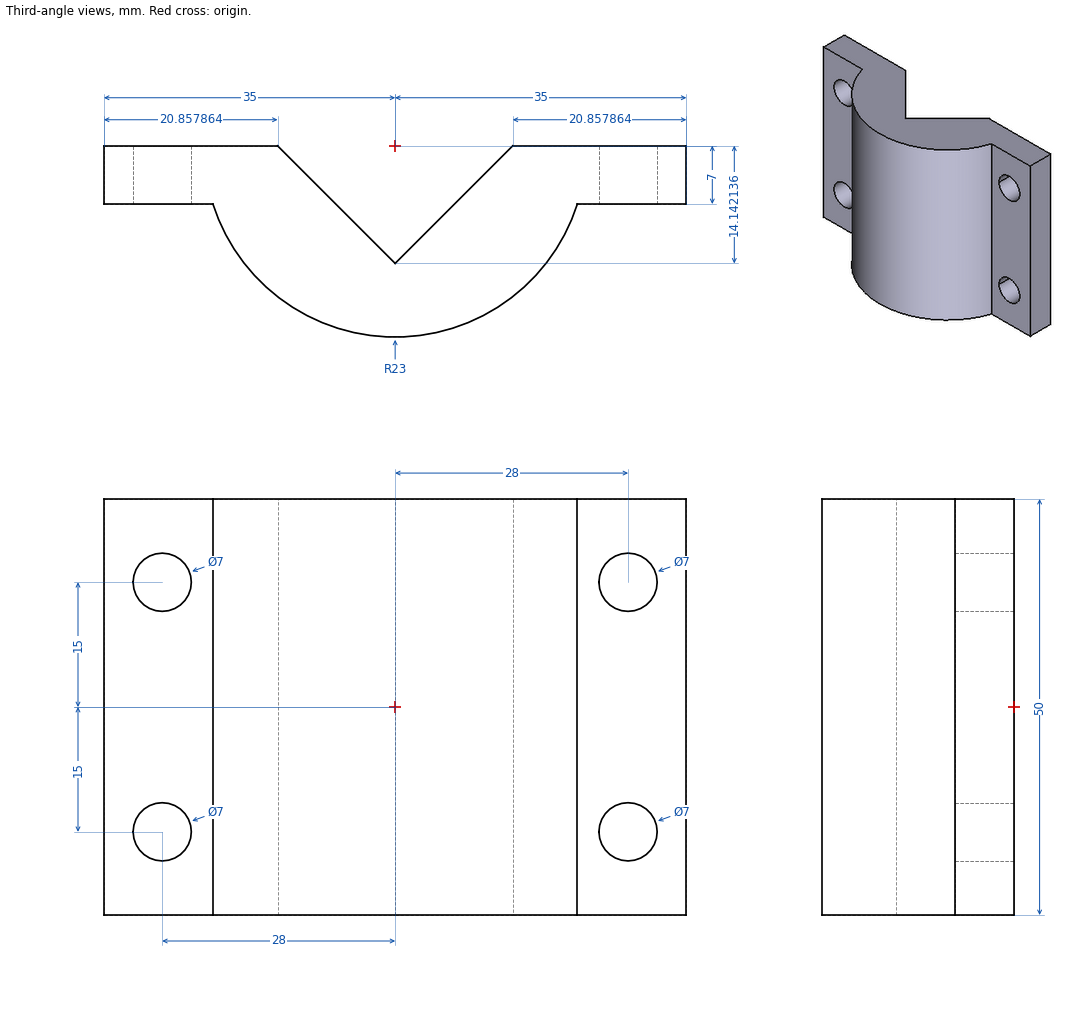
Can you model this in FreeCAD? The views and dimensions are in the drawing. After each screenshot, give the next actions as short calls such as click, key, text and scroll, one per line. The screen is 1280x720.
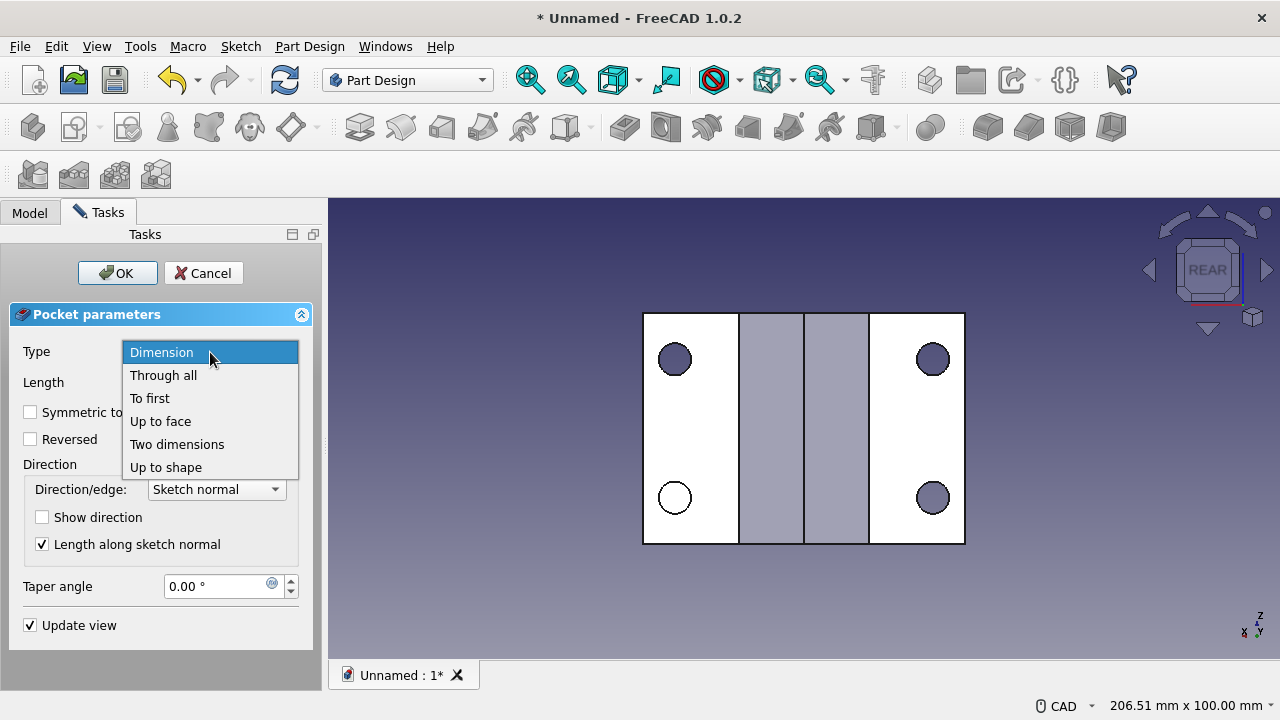
click(208, 398)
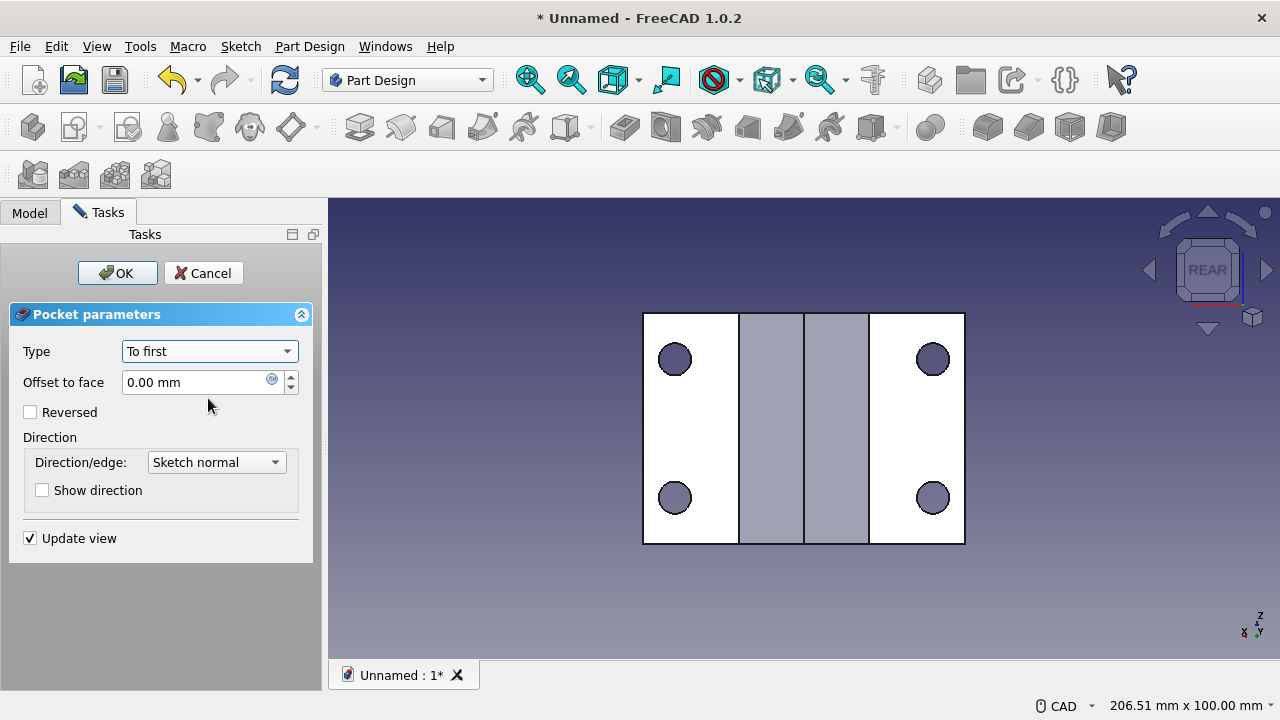
click(118, 273)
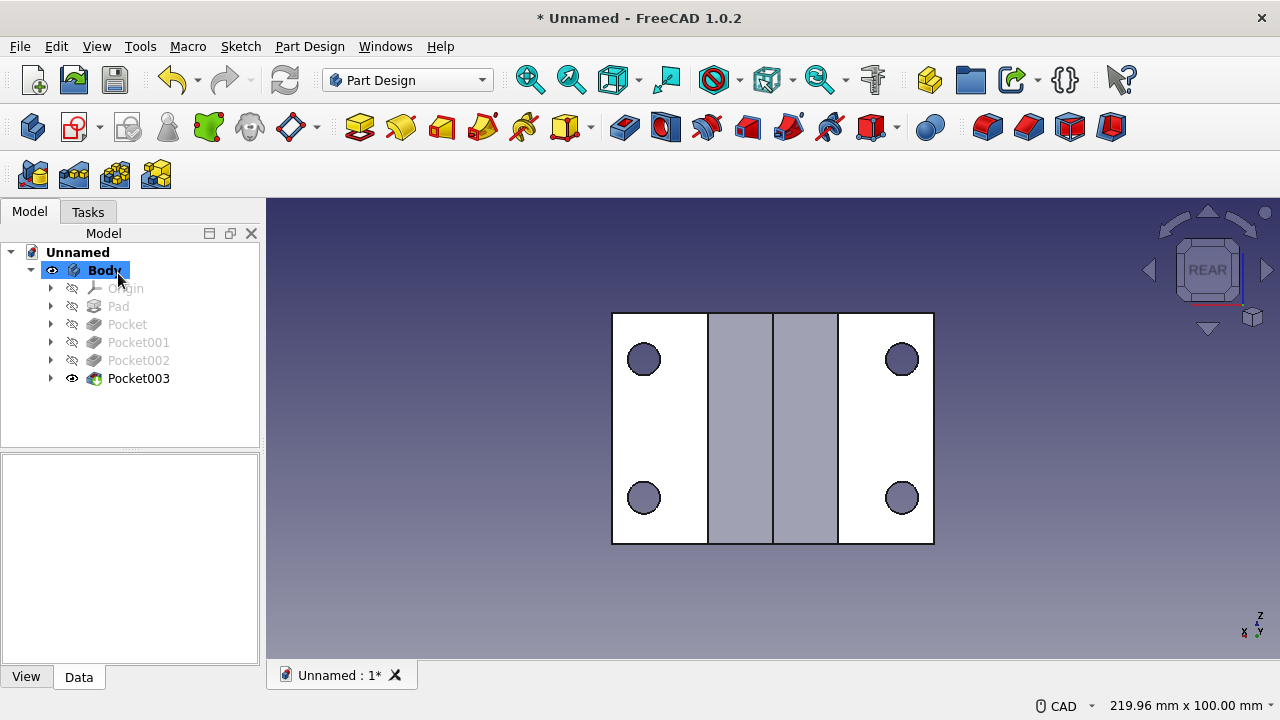
key(0)